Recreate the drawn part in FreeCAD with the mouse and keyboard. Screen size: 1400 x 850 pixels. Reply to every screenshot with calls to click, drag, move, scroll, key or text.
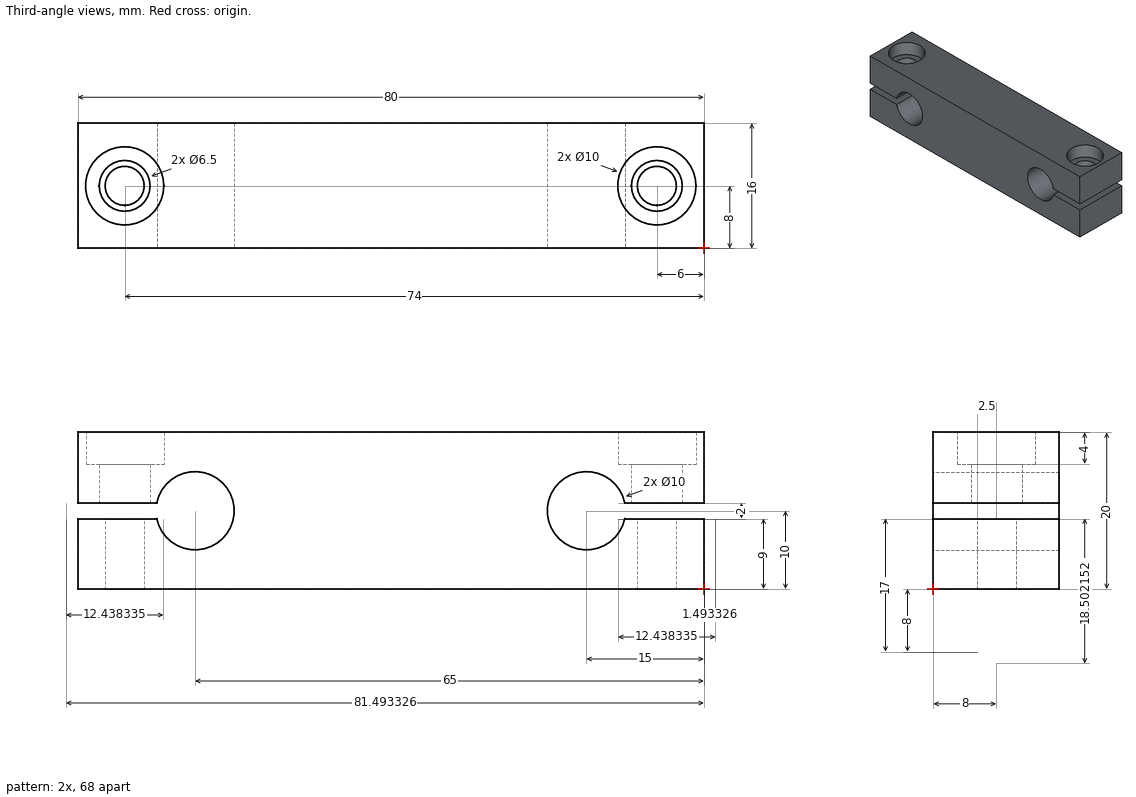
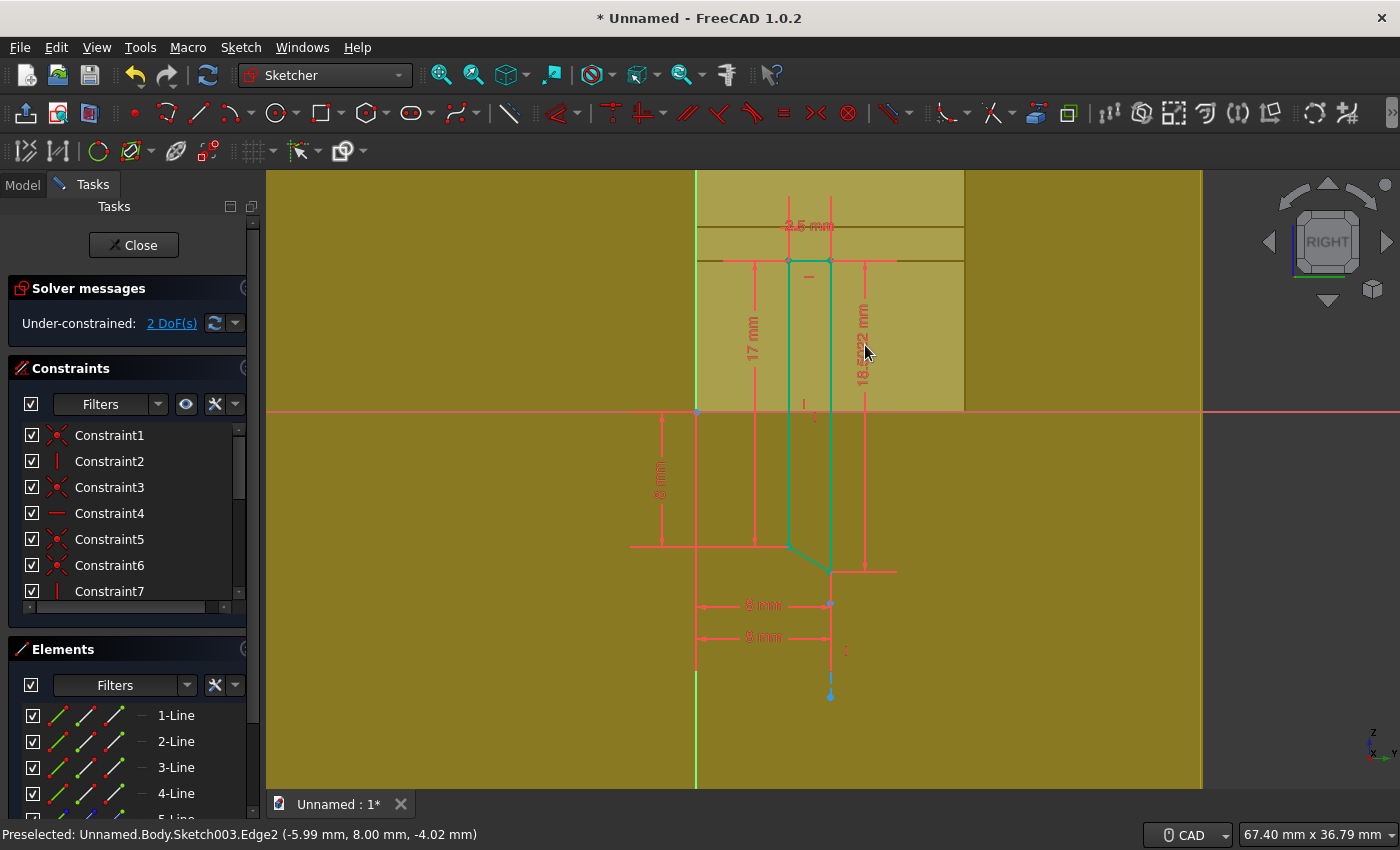
click(134, 245)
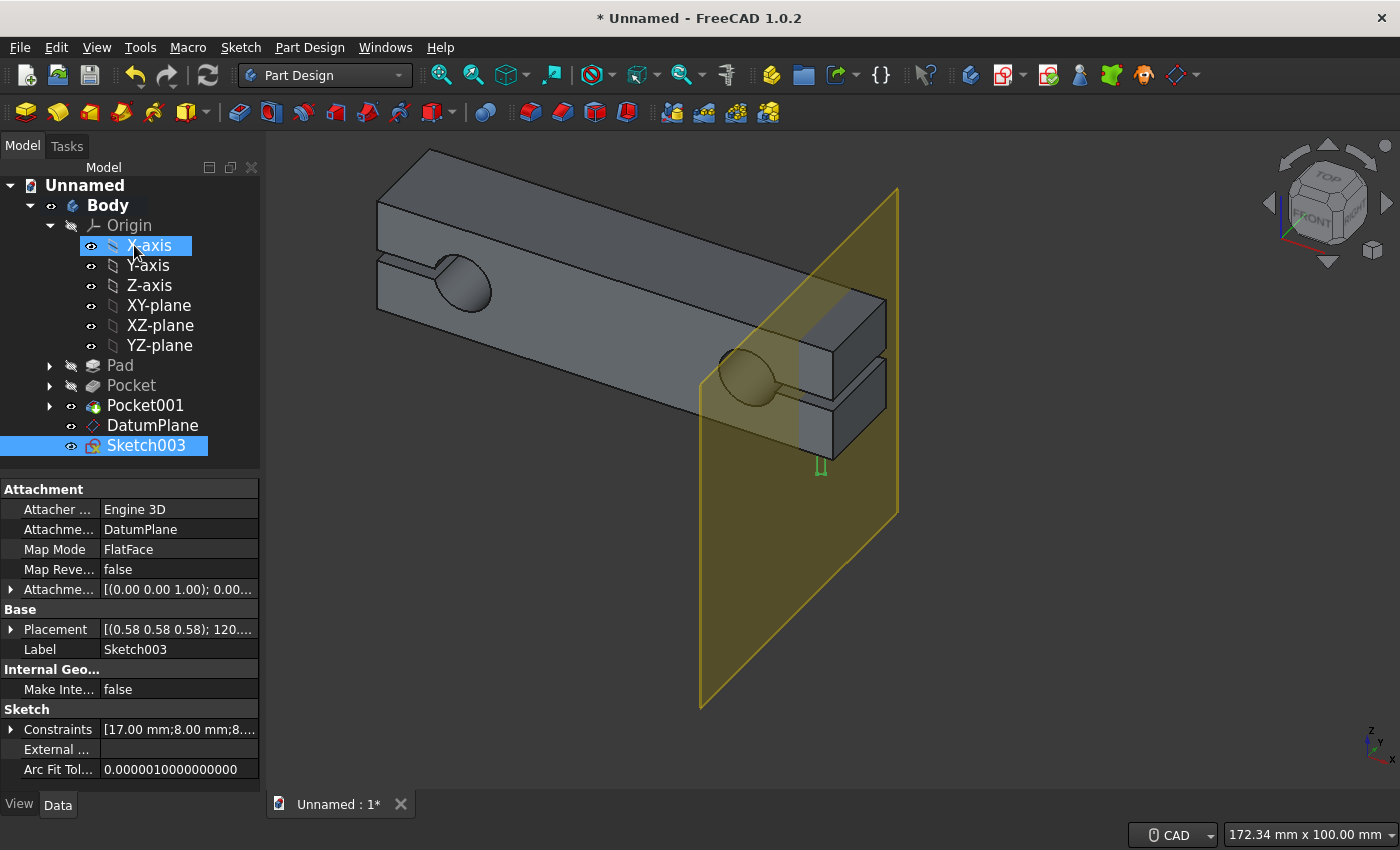
click(304, 112)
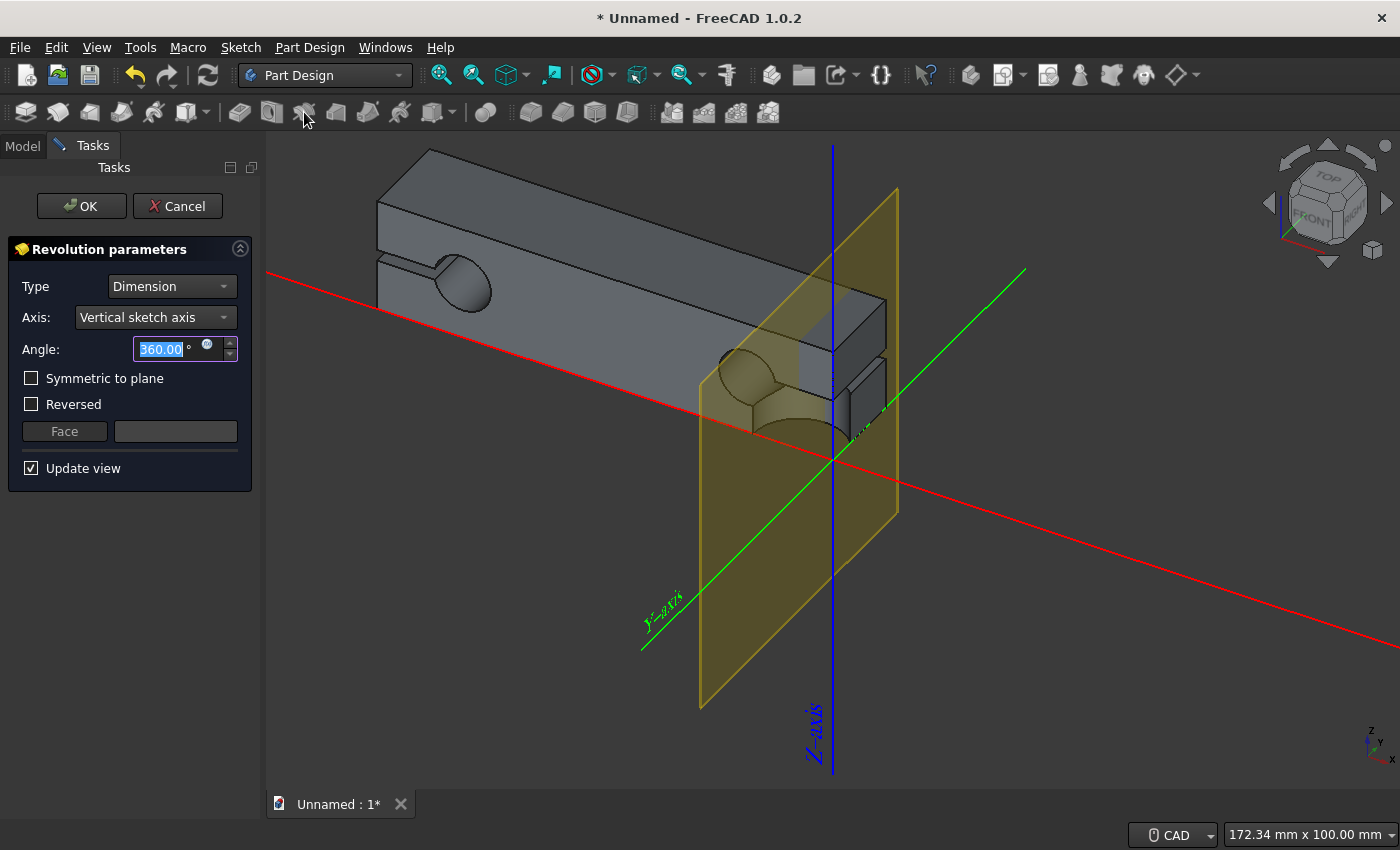
click(156, 318)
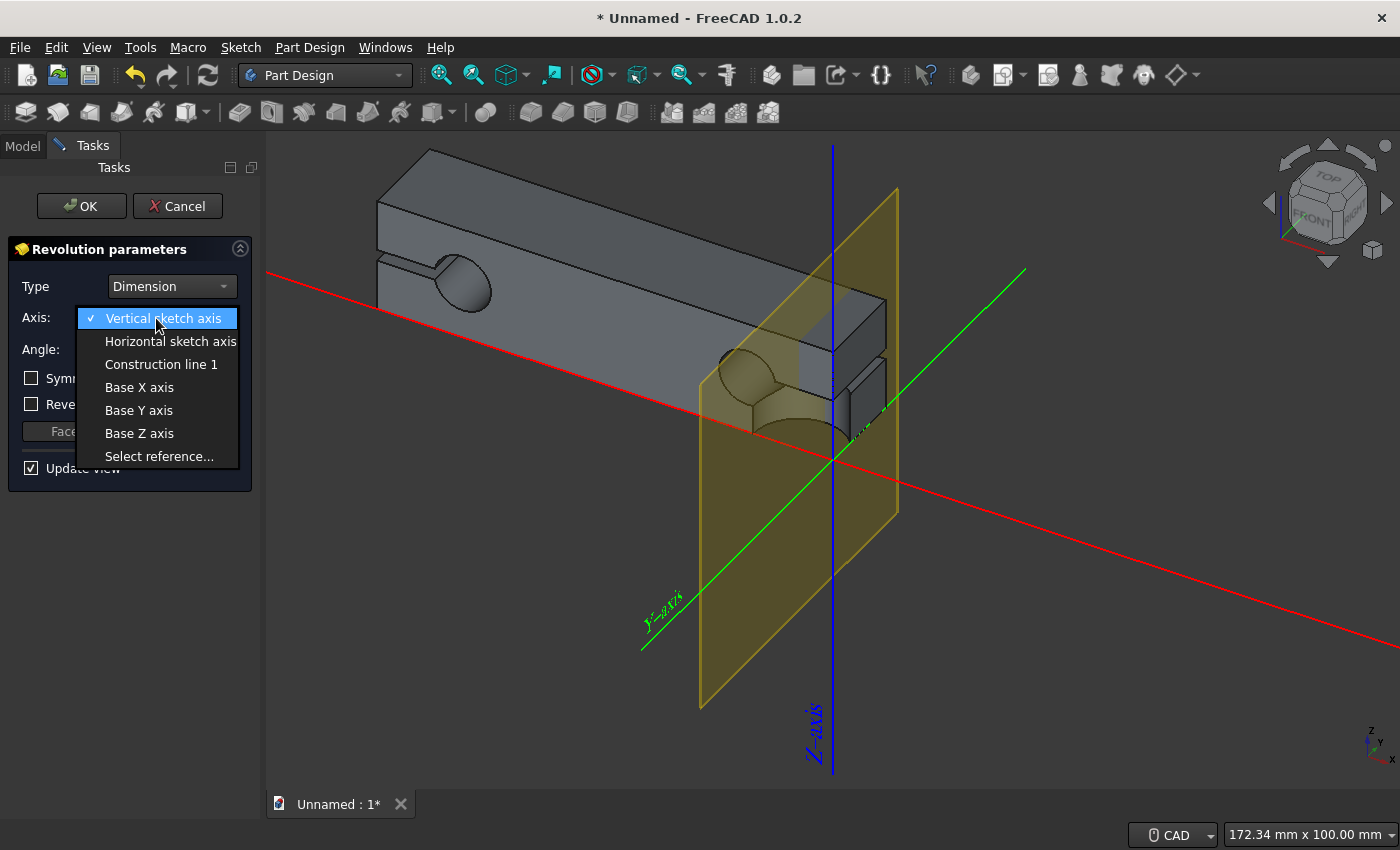
click(156, 364)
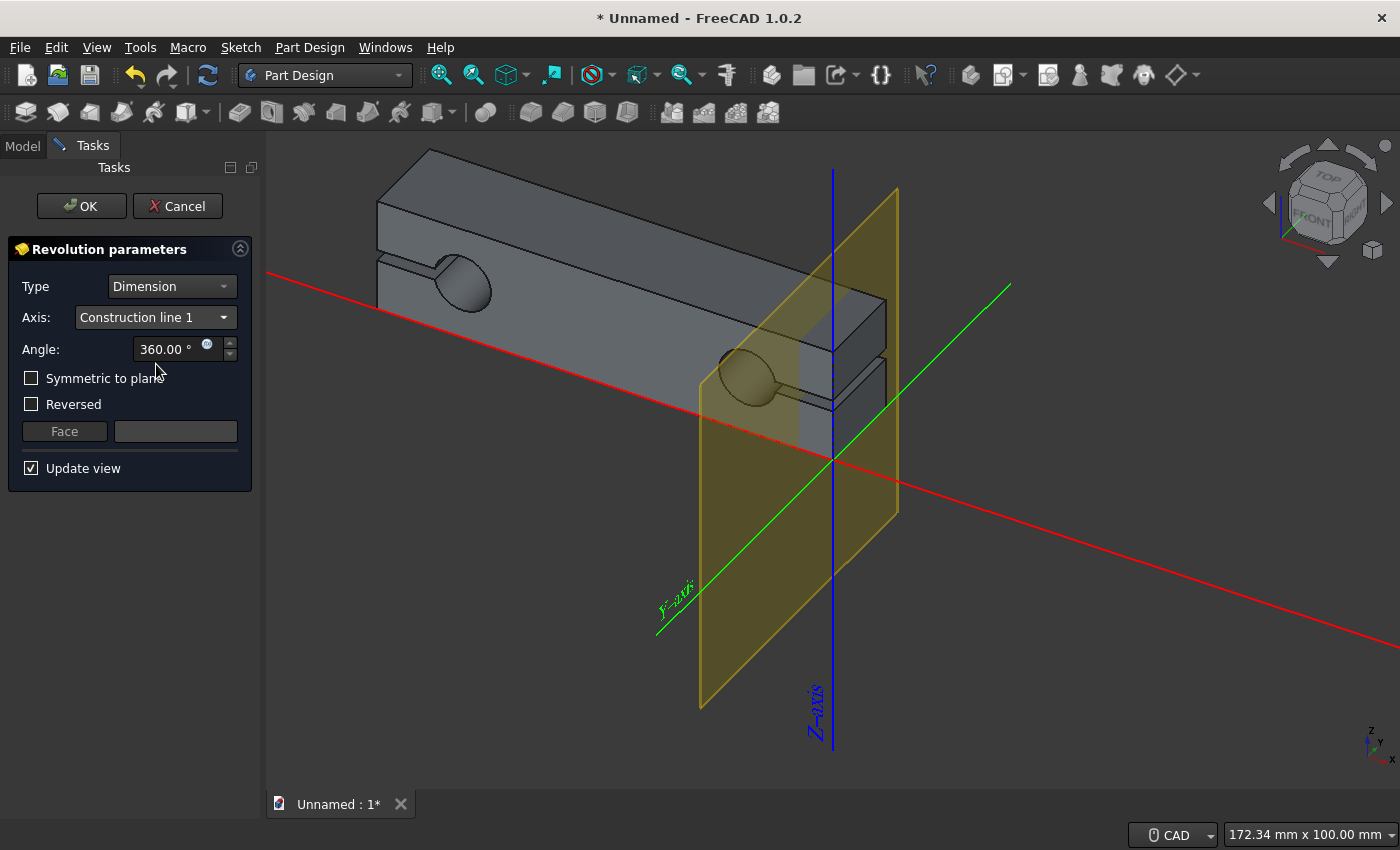
click(82, 206)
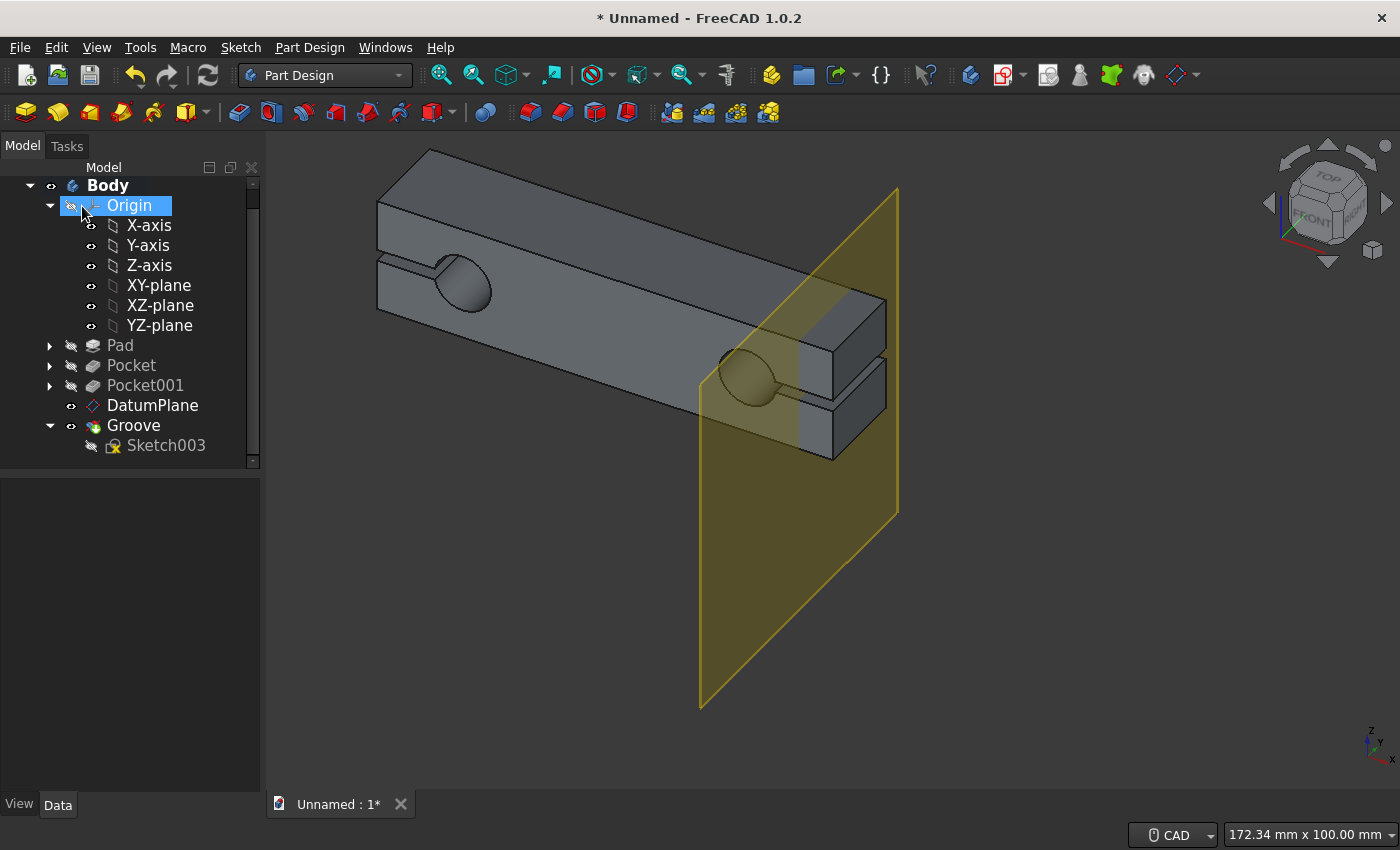
click(116, 406)
key(space)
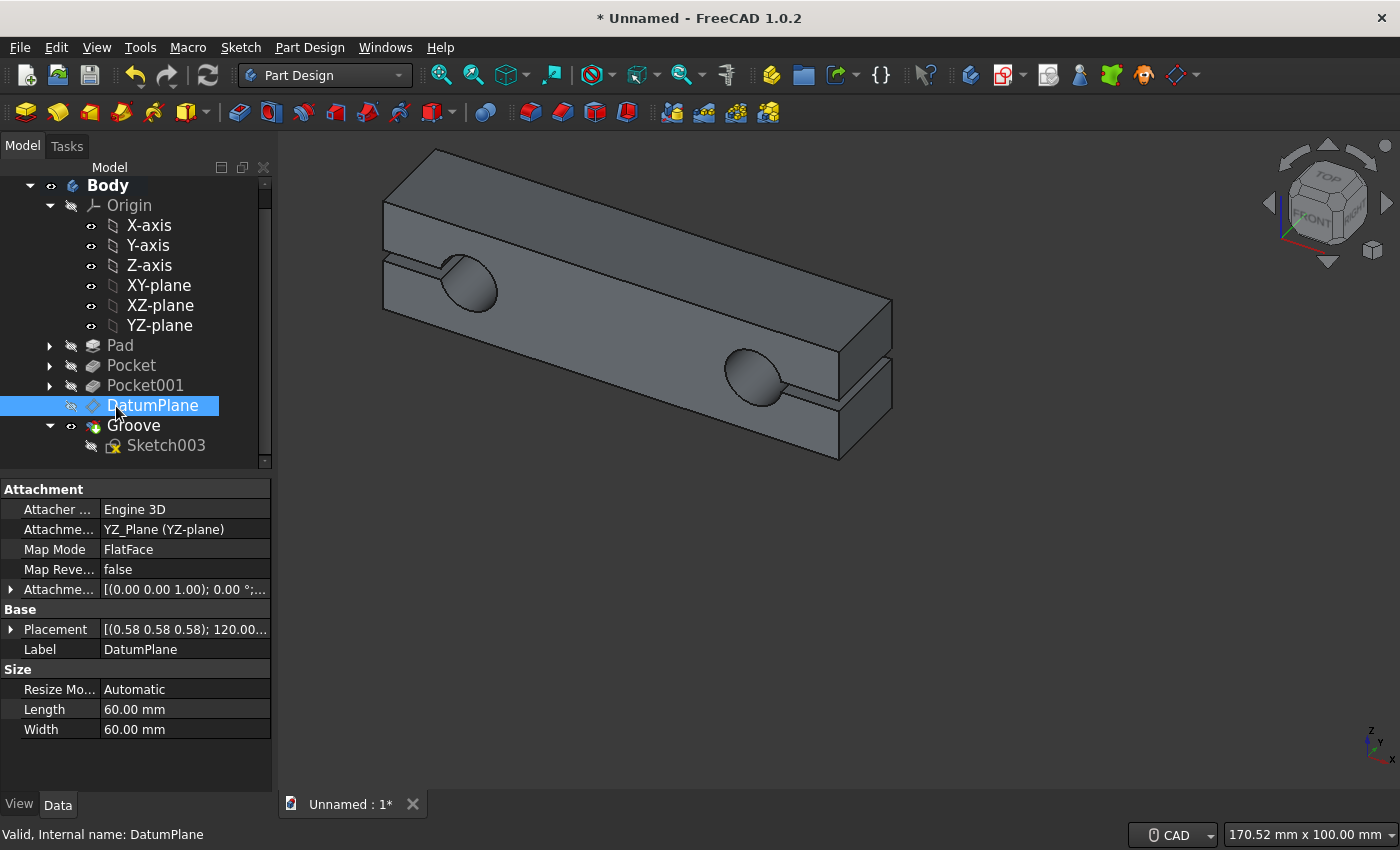
click(116, 426)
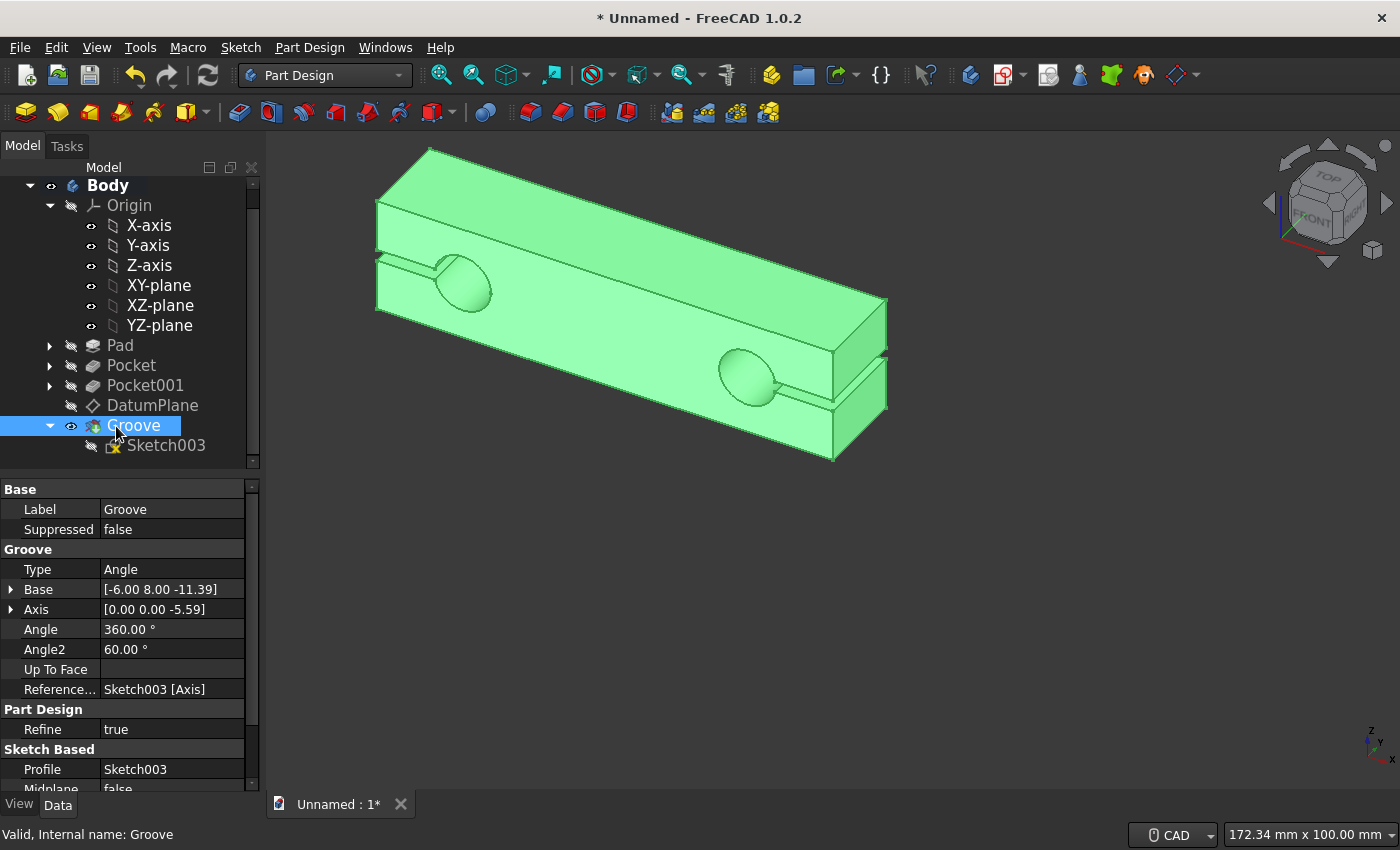
click(704, 112)